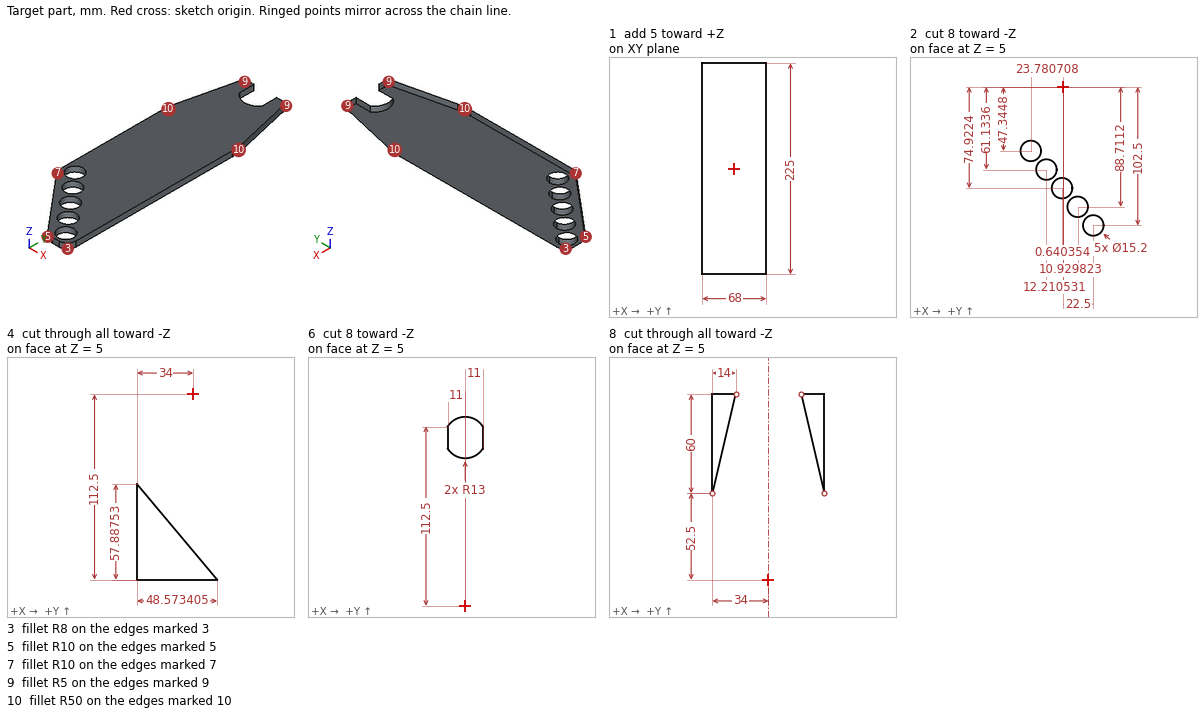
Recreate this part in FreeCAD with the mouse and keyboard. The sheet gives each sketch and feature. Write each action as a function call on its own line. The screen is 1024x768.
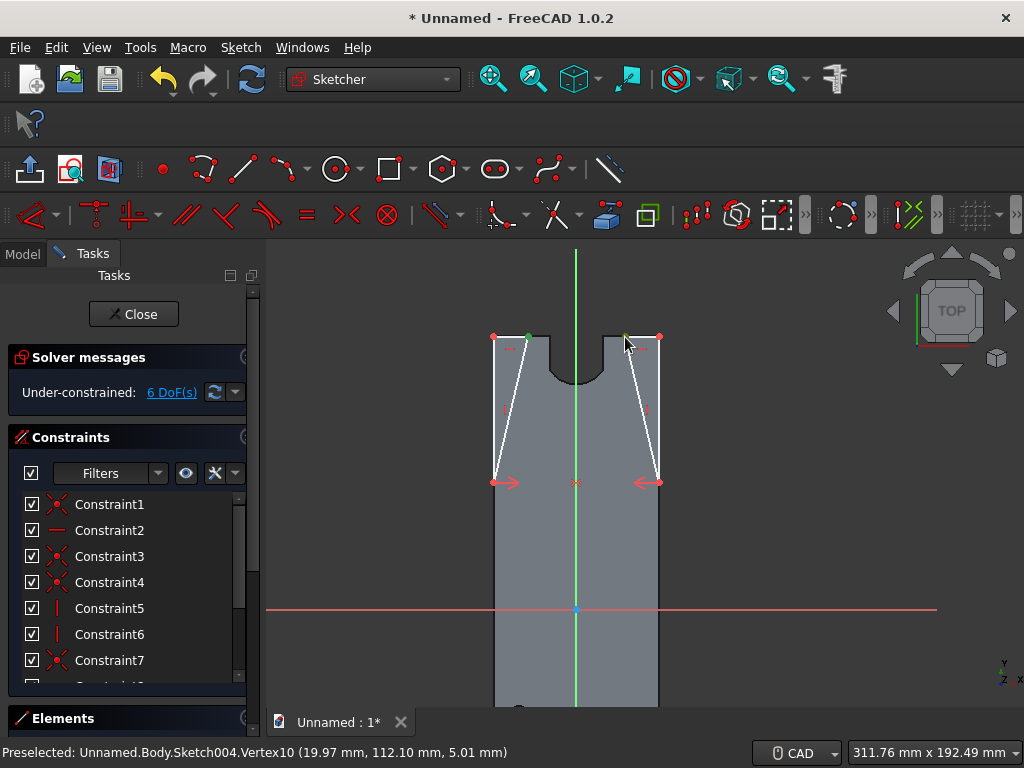
click(576, 650)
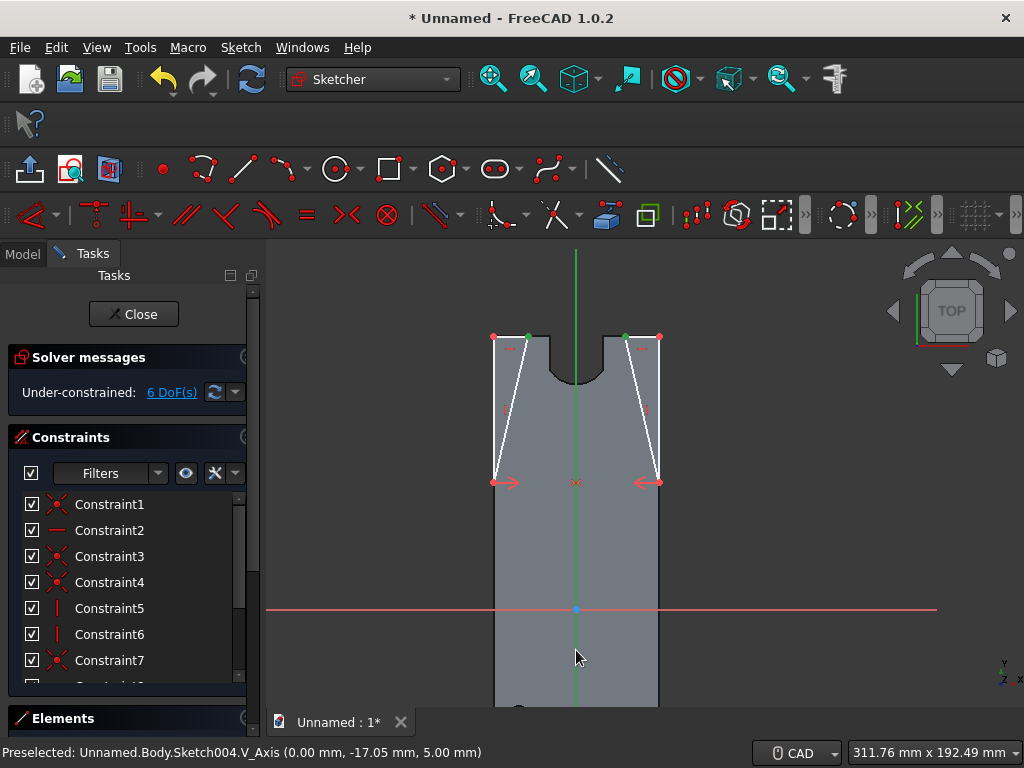
key(s)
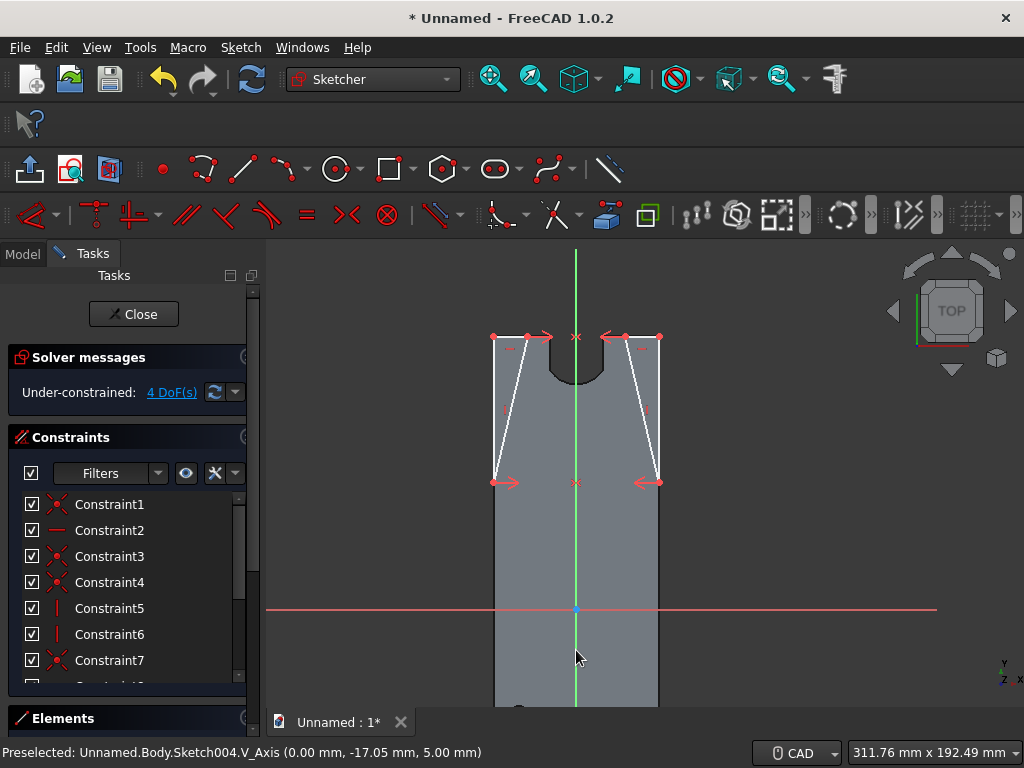
key(d)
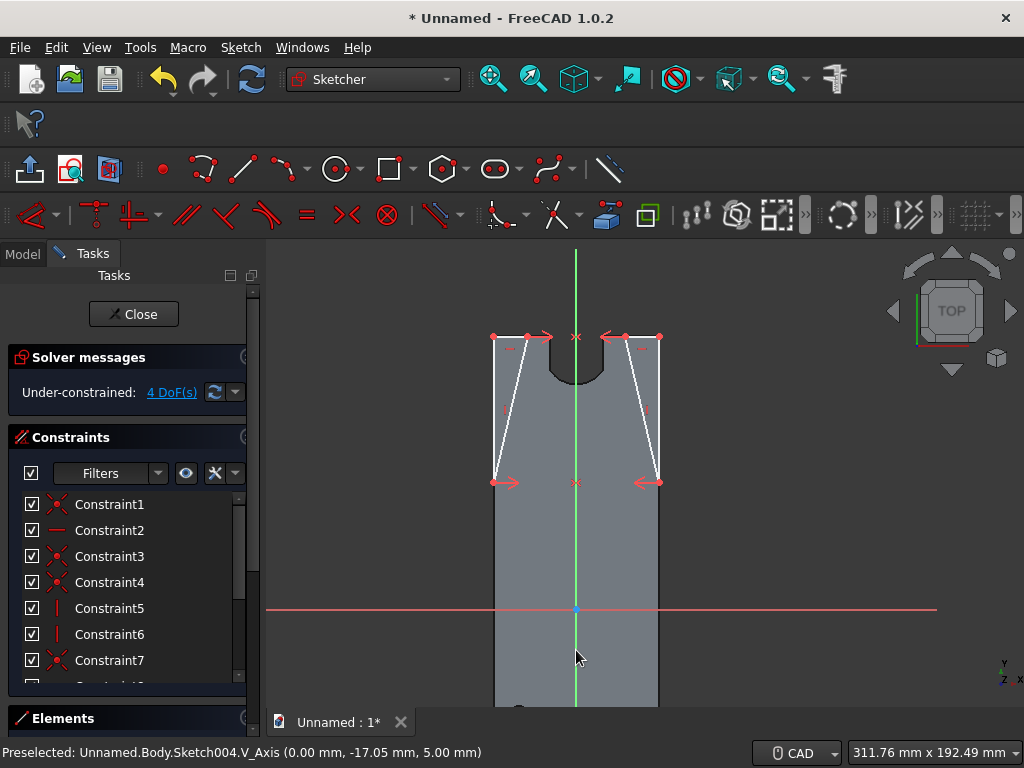
scroll(518, 337, up, 2)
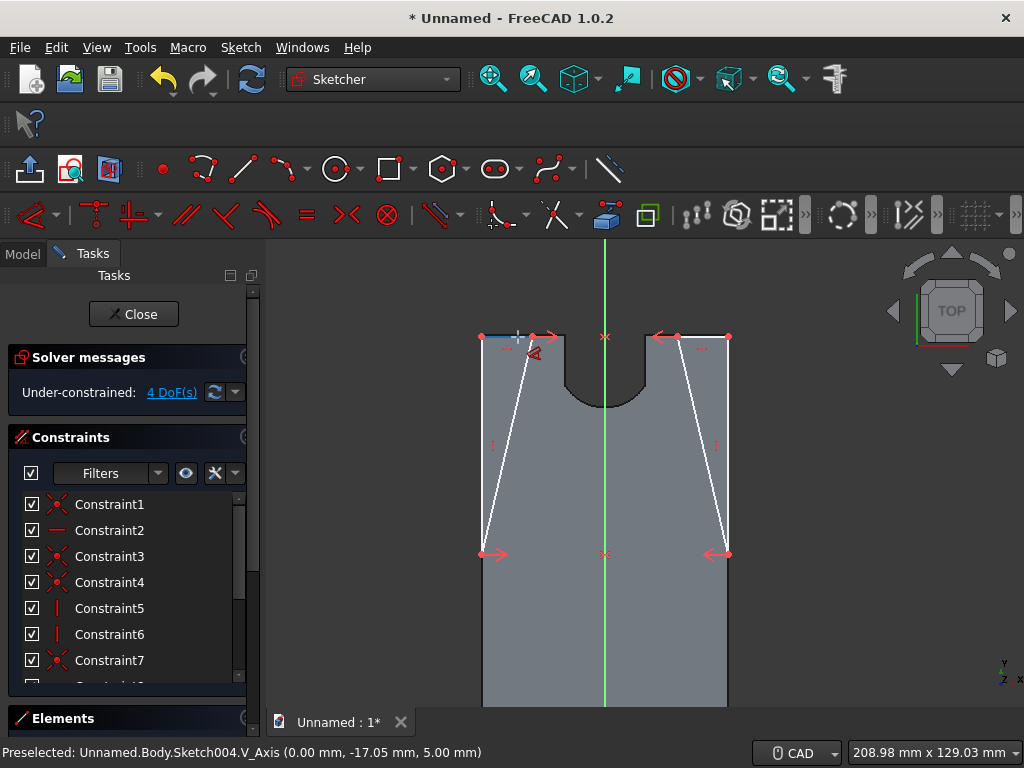
click(517, 337)
click(507, 303)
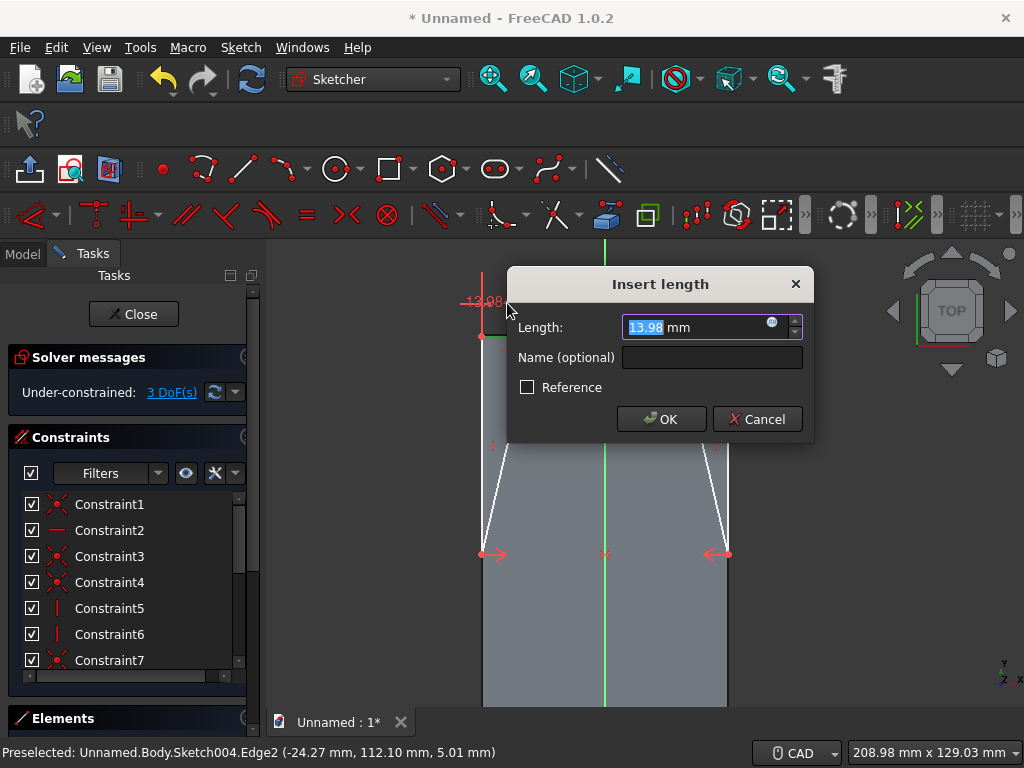
text(14)
key(Return)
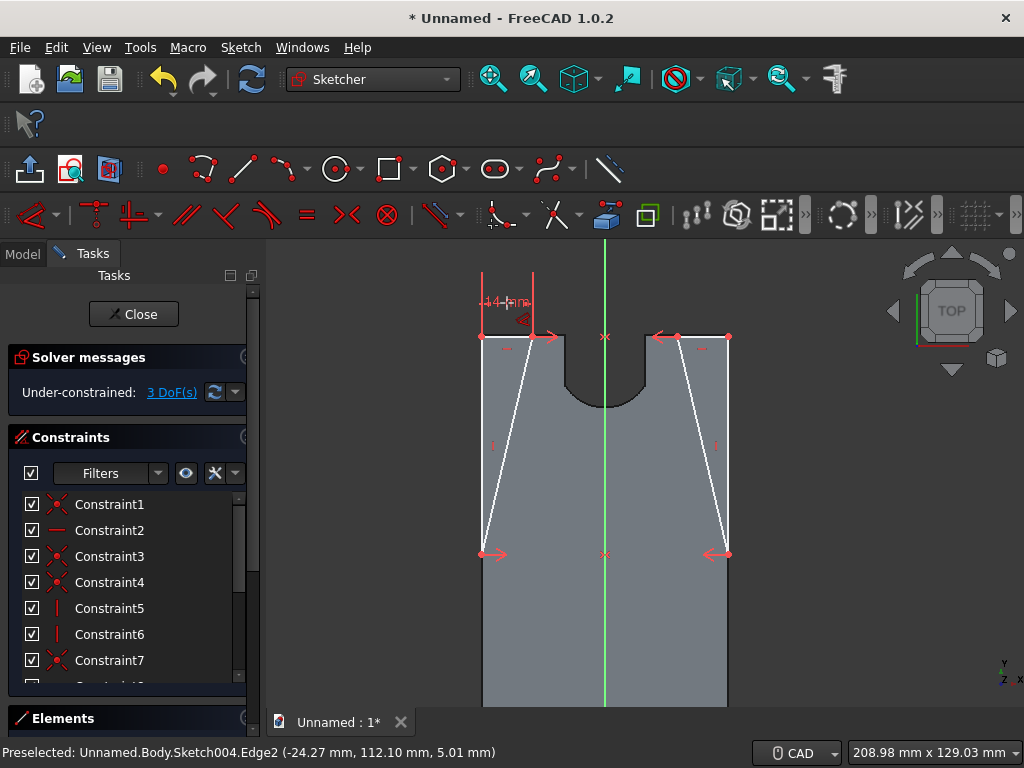
click(482, 402)
click(448, 446)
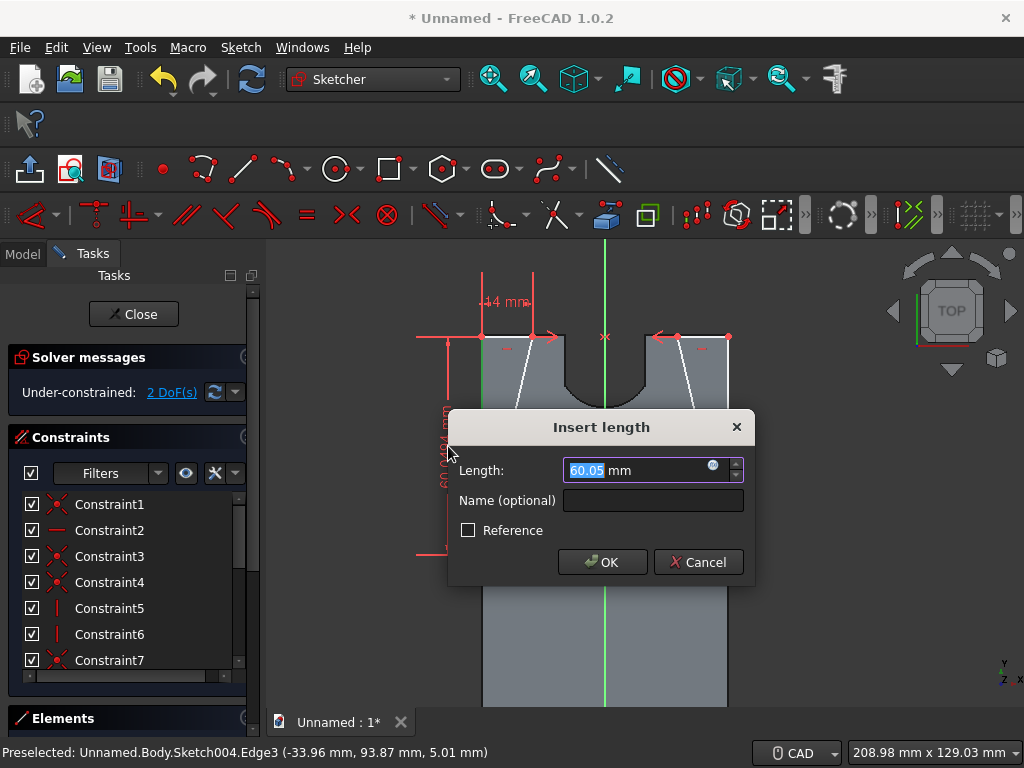
text(60)
key(Return)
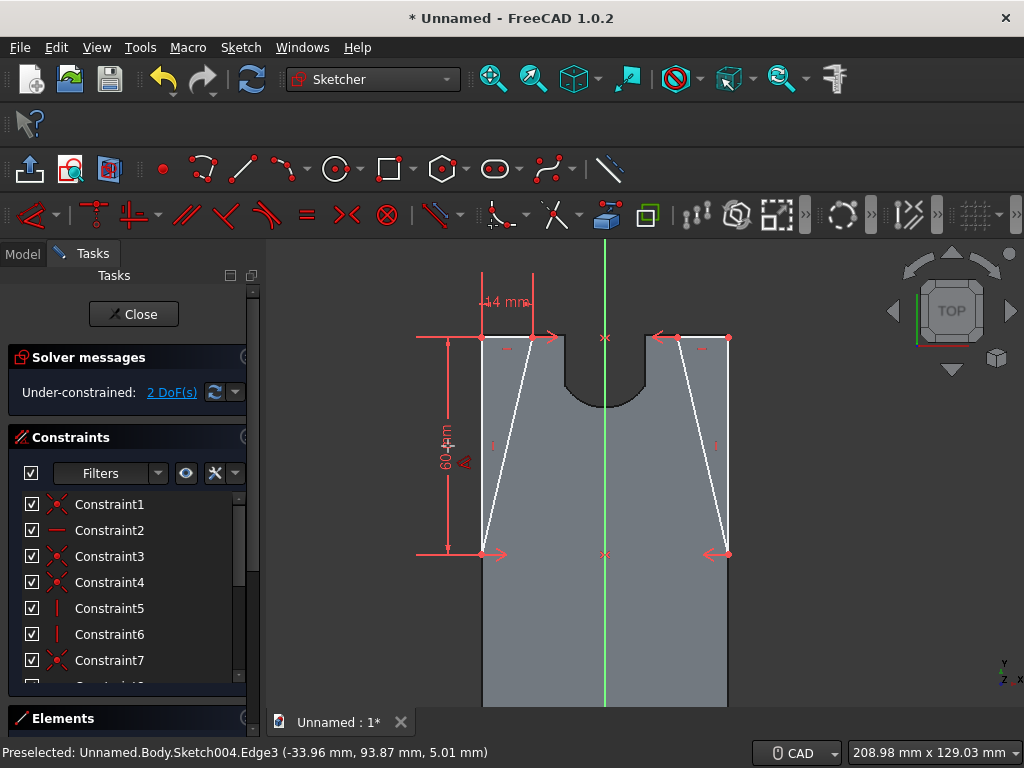
click(482, 555)
click(543, 521)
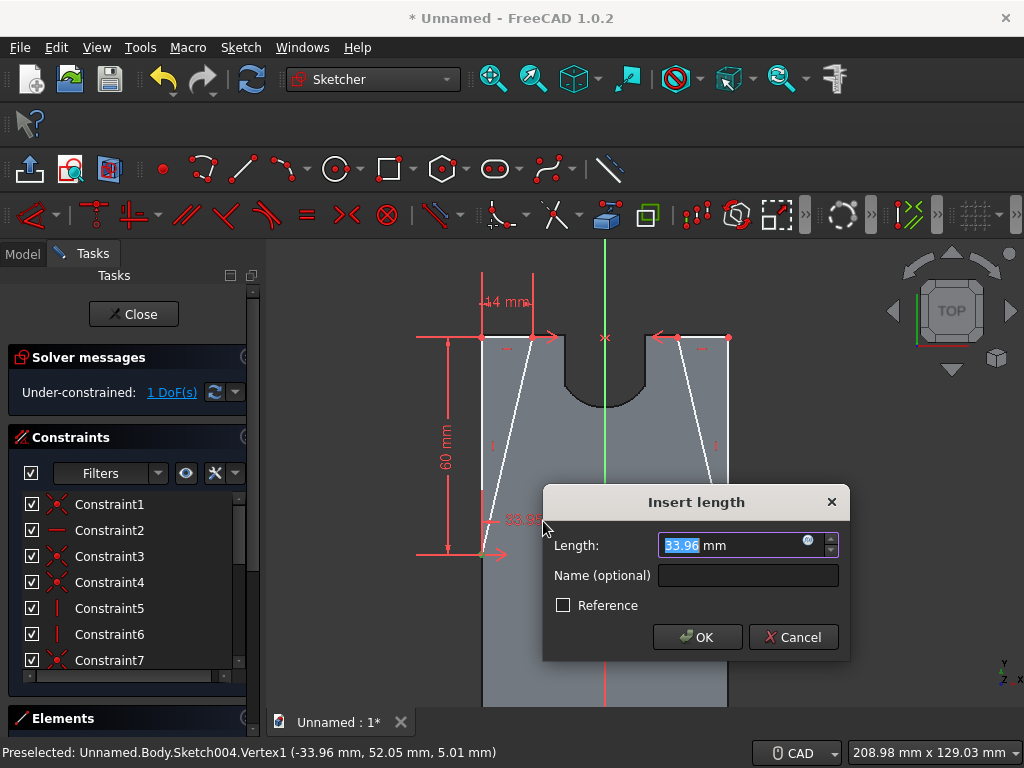
text(34)
key(Return)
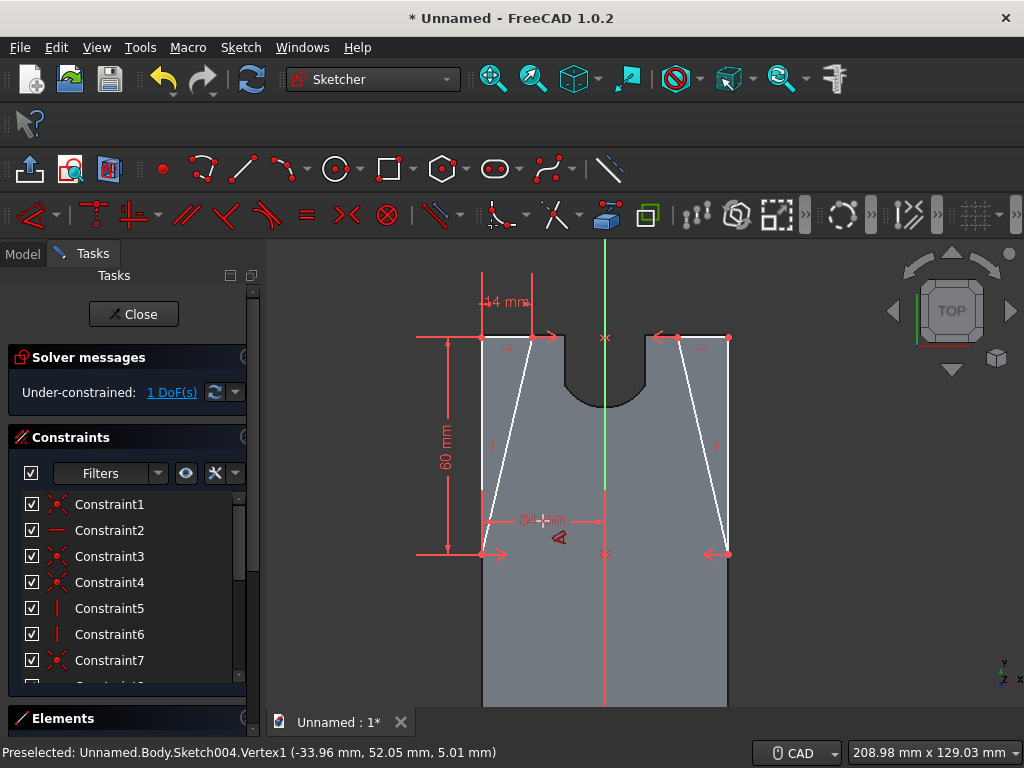
click(482, 555)
click(448, 617)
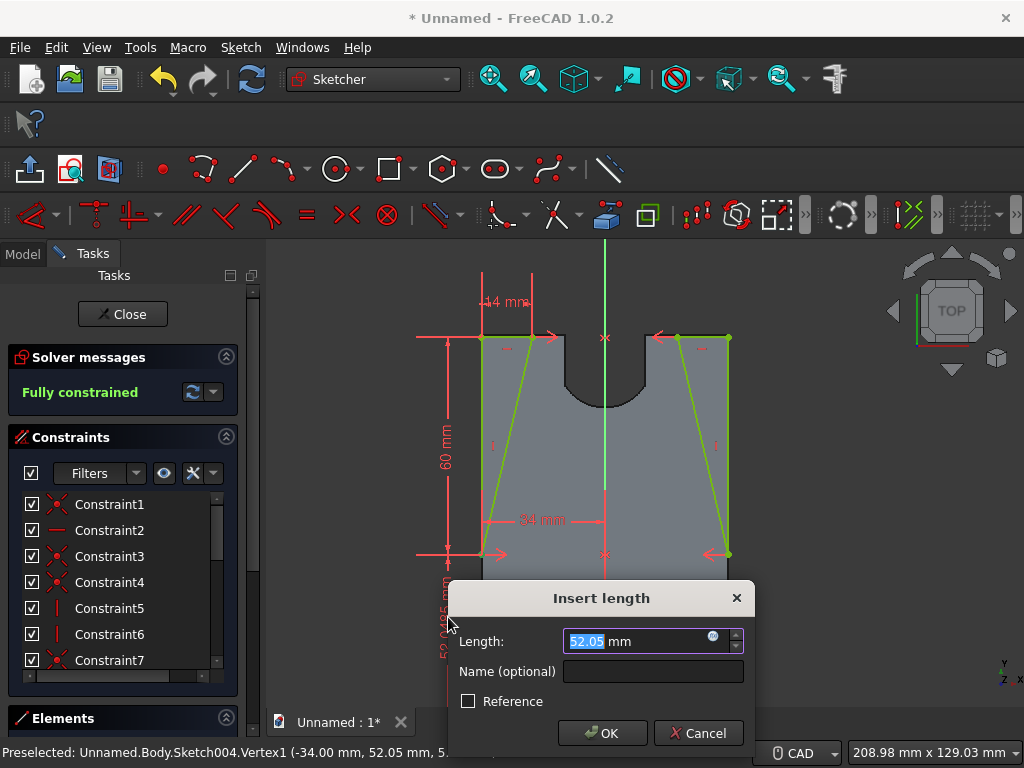
text(52.5)
key(Return)
key(Escape)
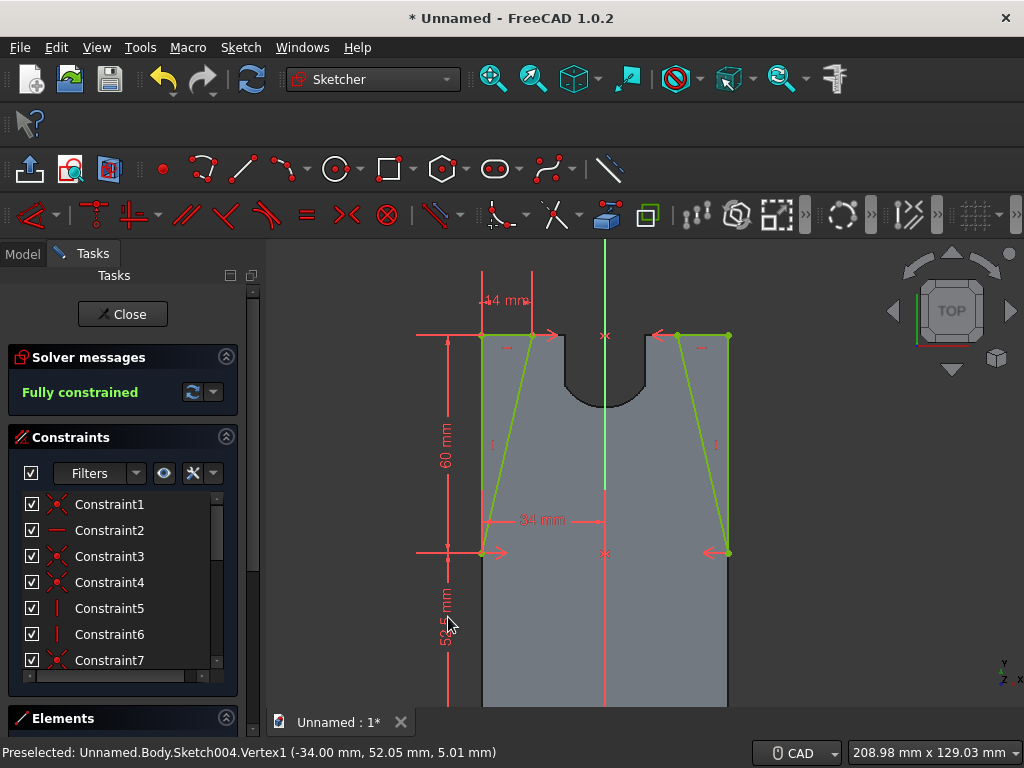
click(123, 314)